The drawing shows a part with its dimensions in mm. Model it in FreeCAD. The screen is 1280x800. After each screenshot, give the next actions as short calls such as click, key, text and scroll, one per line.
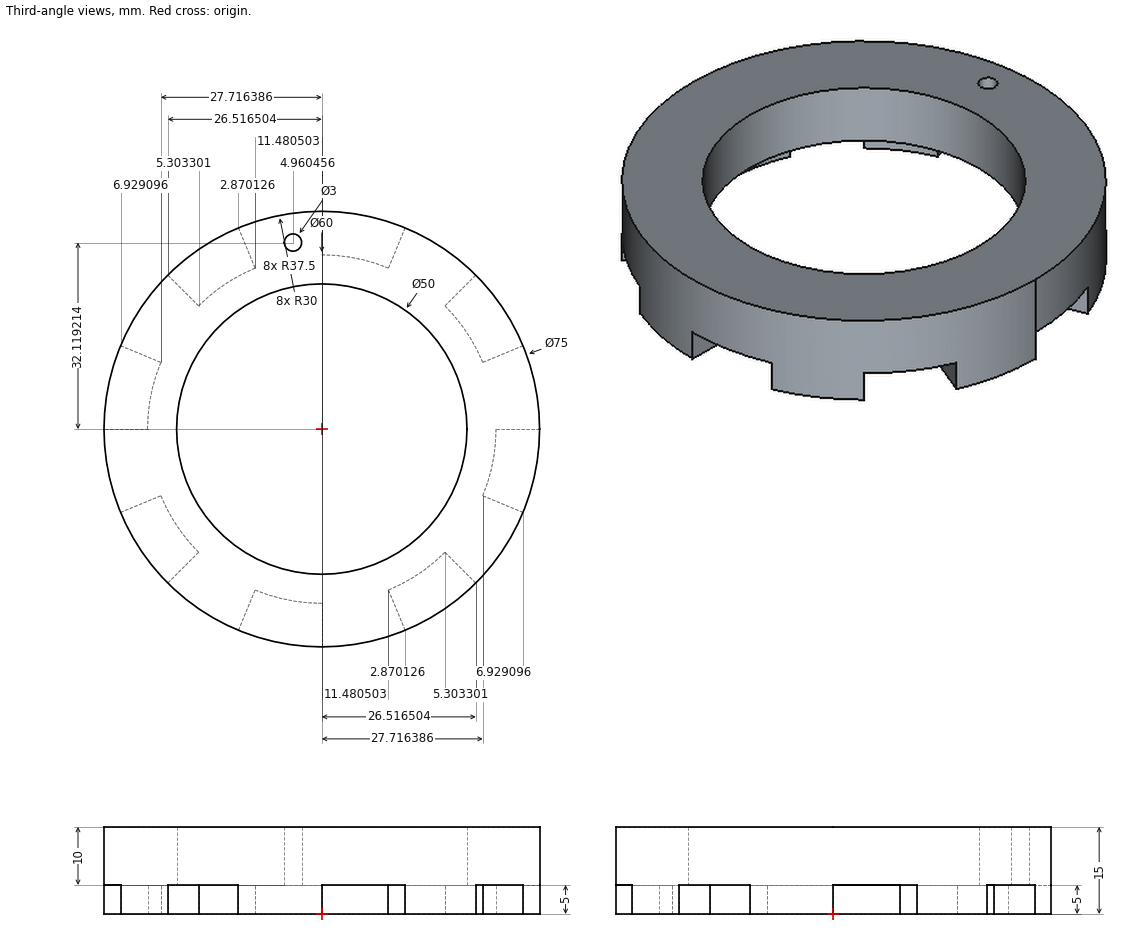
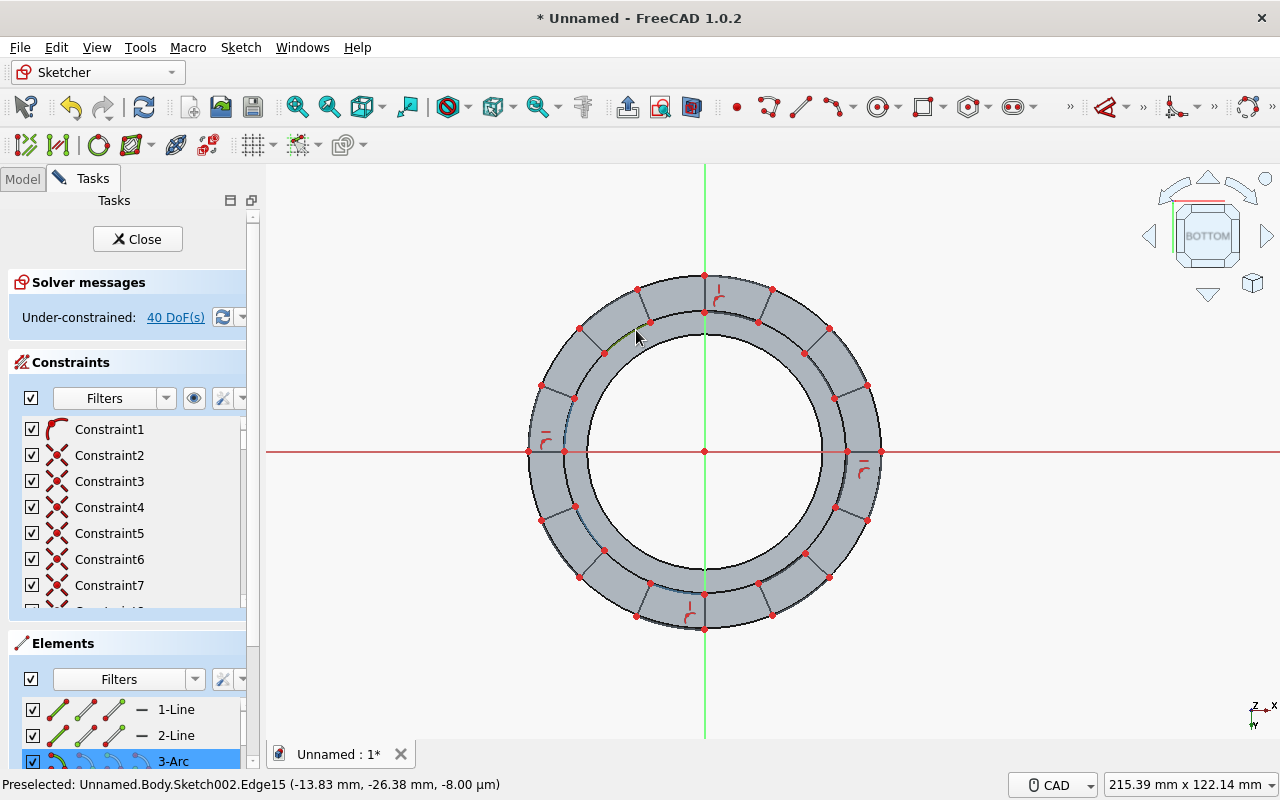
click(743, 318)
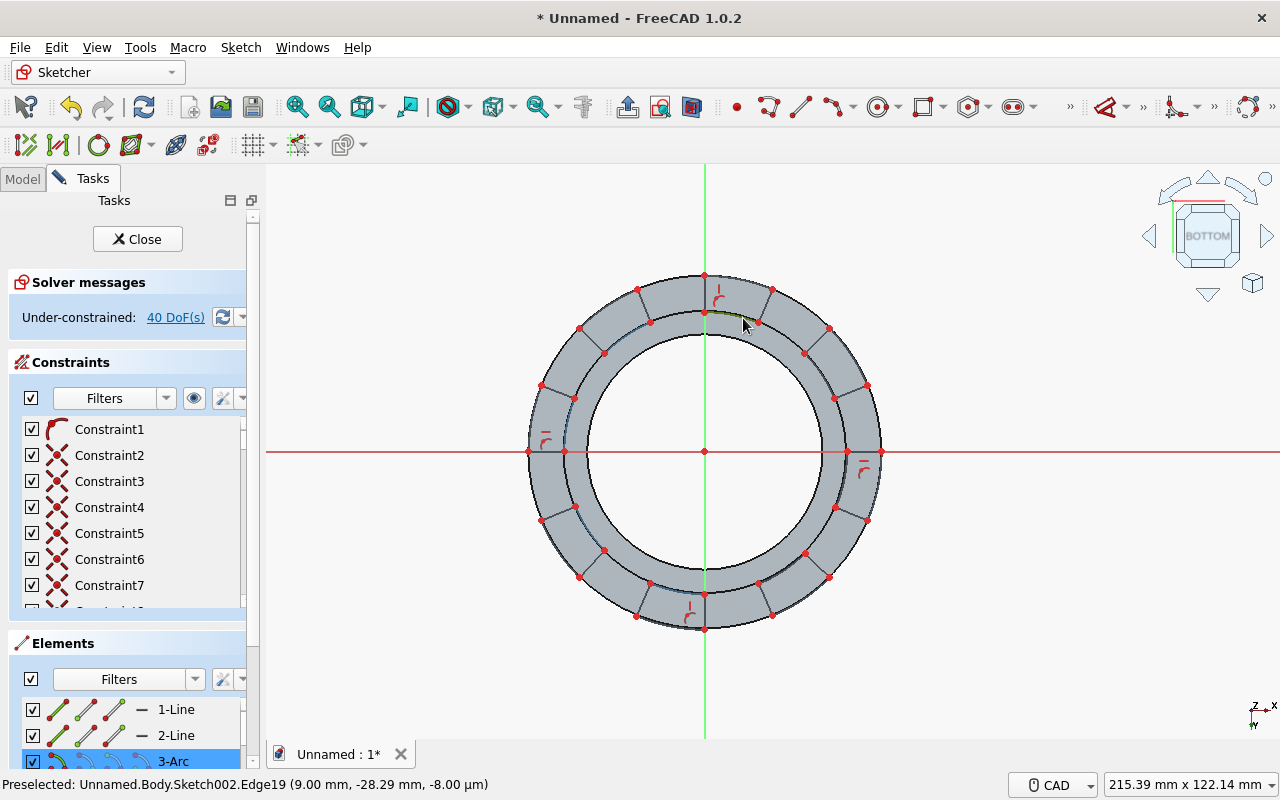
click(827, 384)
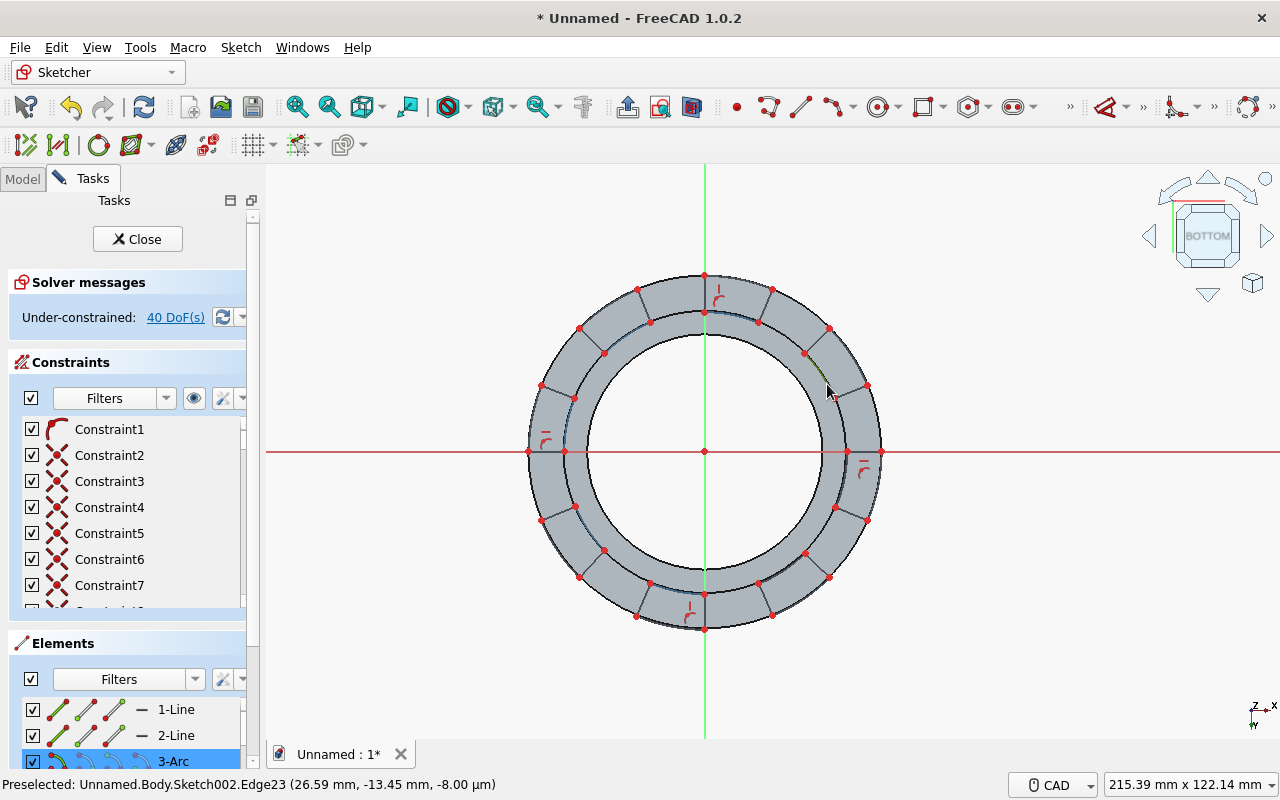
click(841, 491)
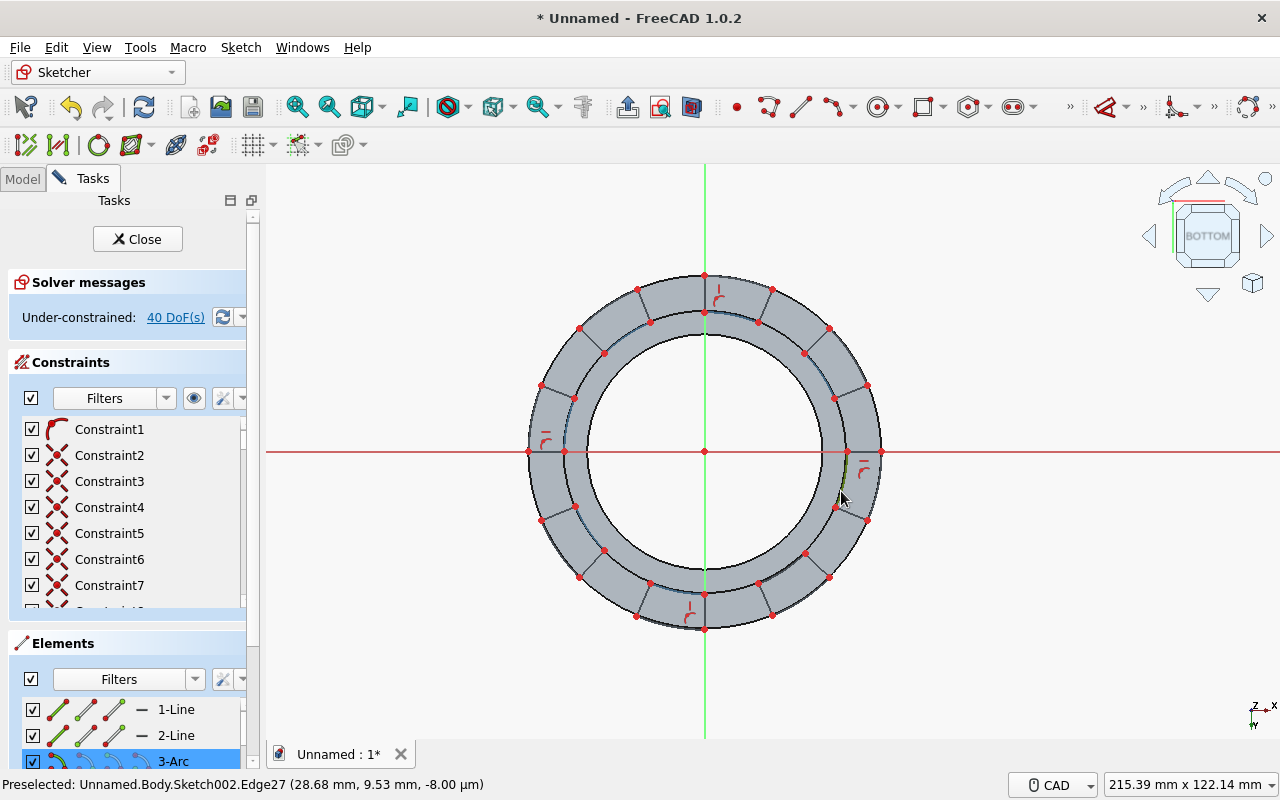
click(774, 577)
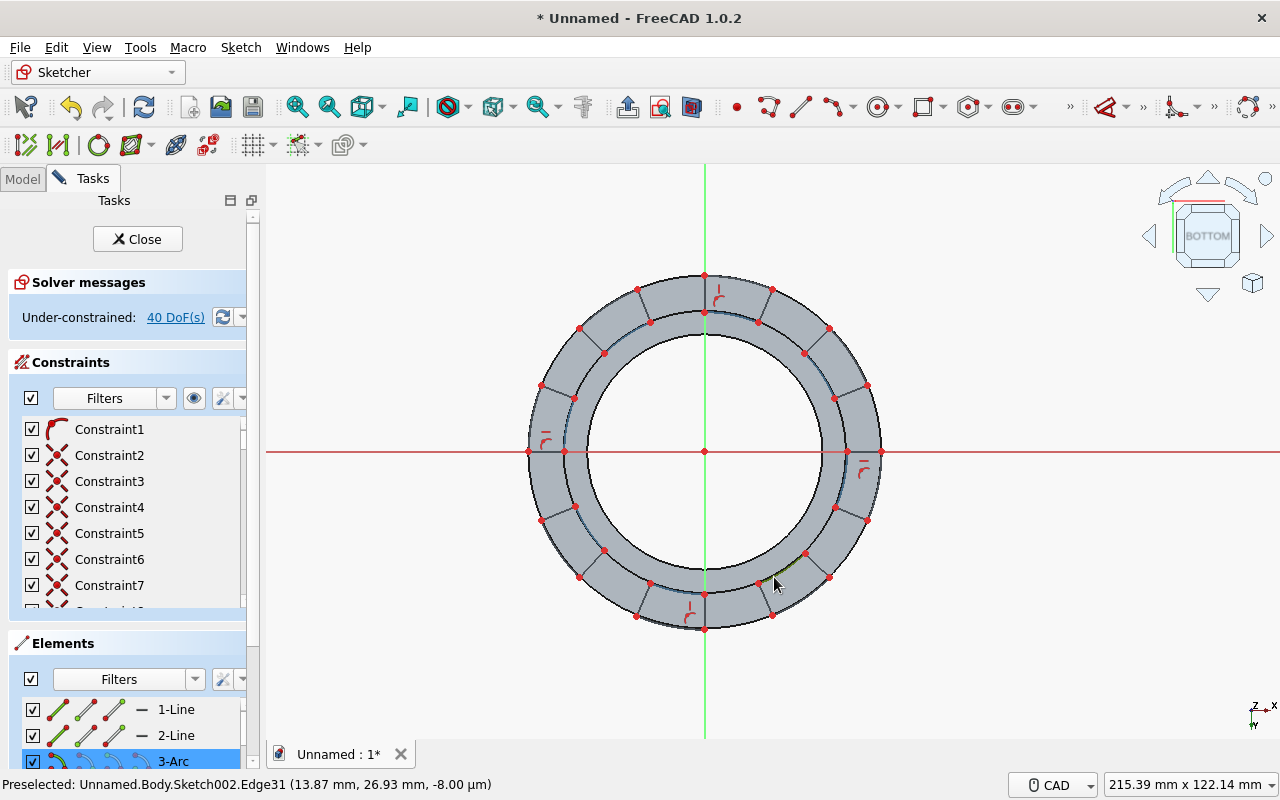
key(e)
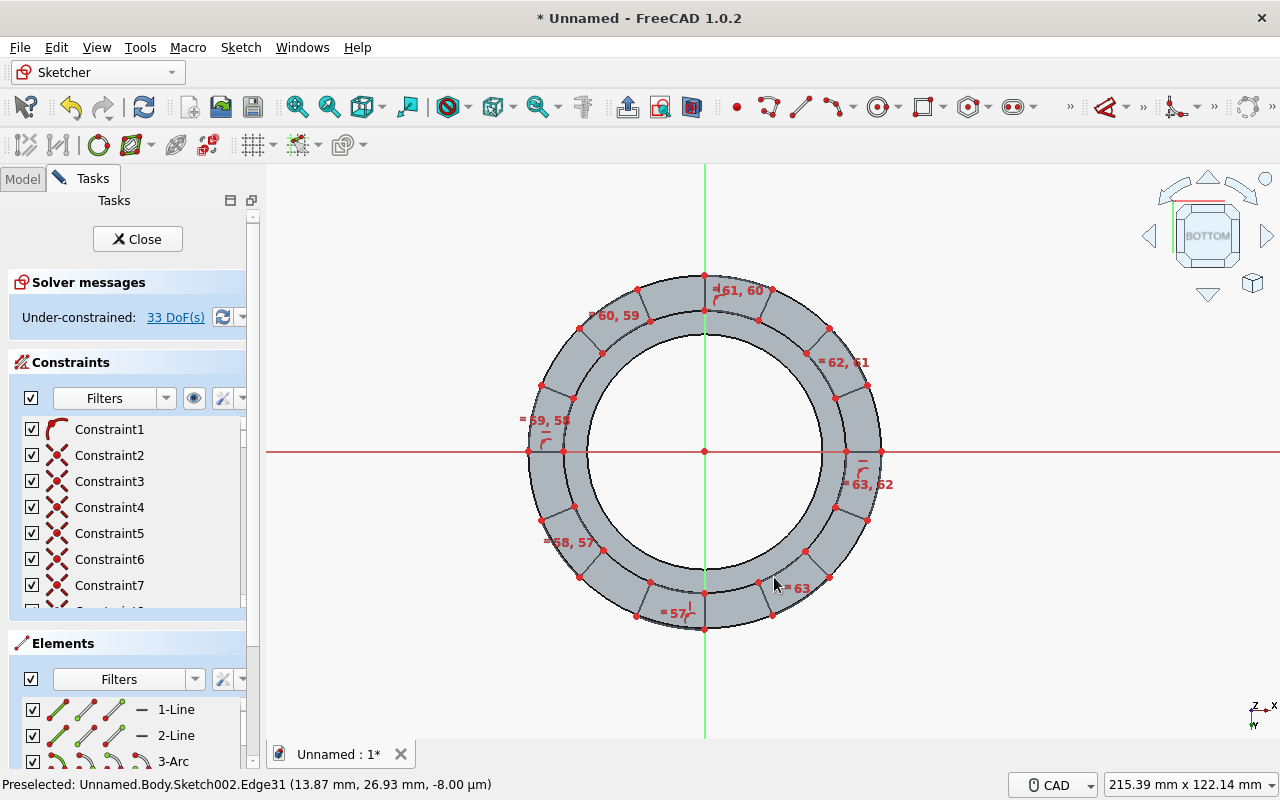
click(657, 623)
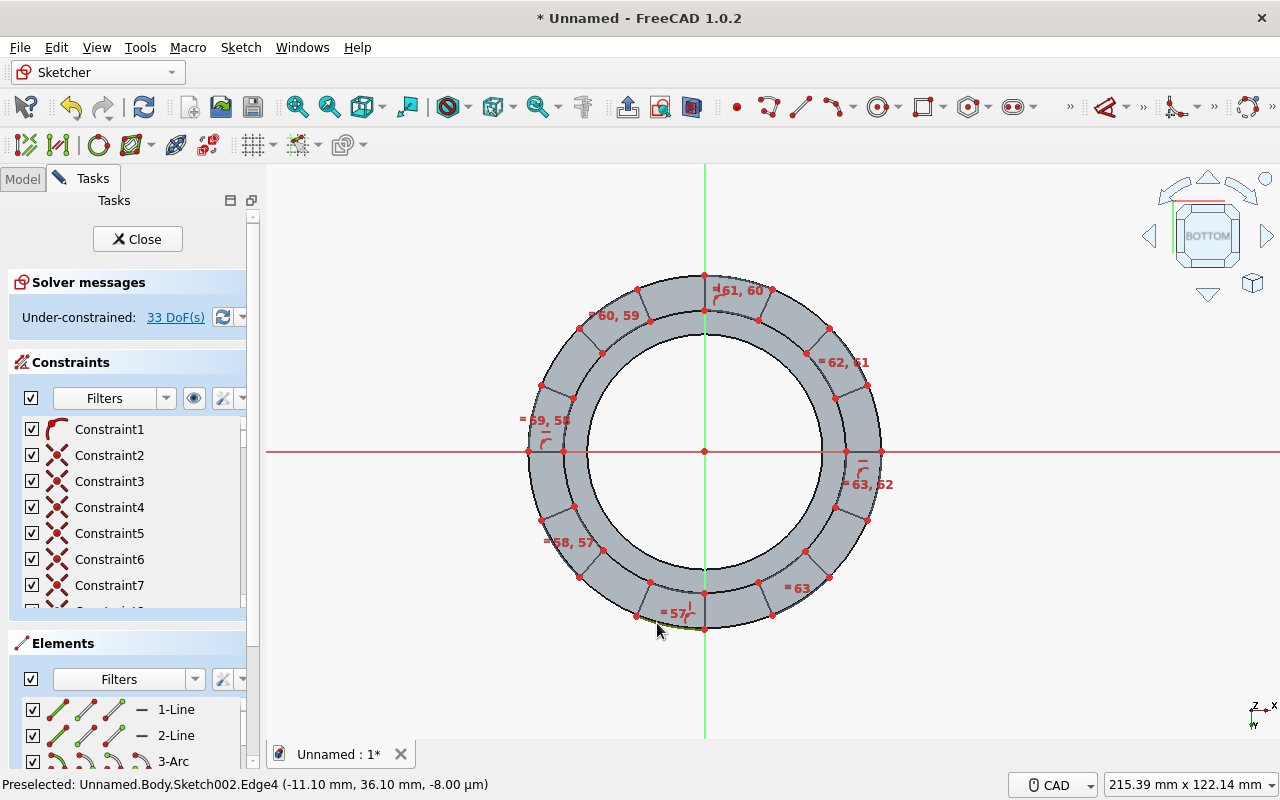
click(566, 562)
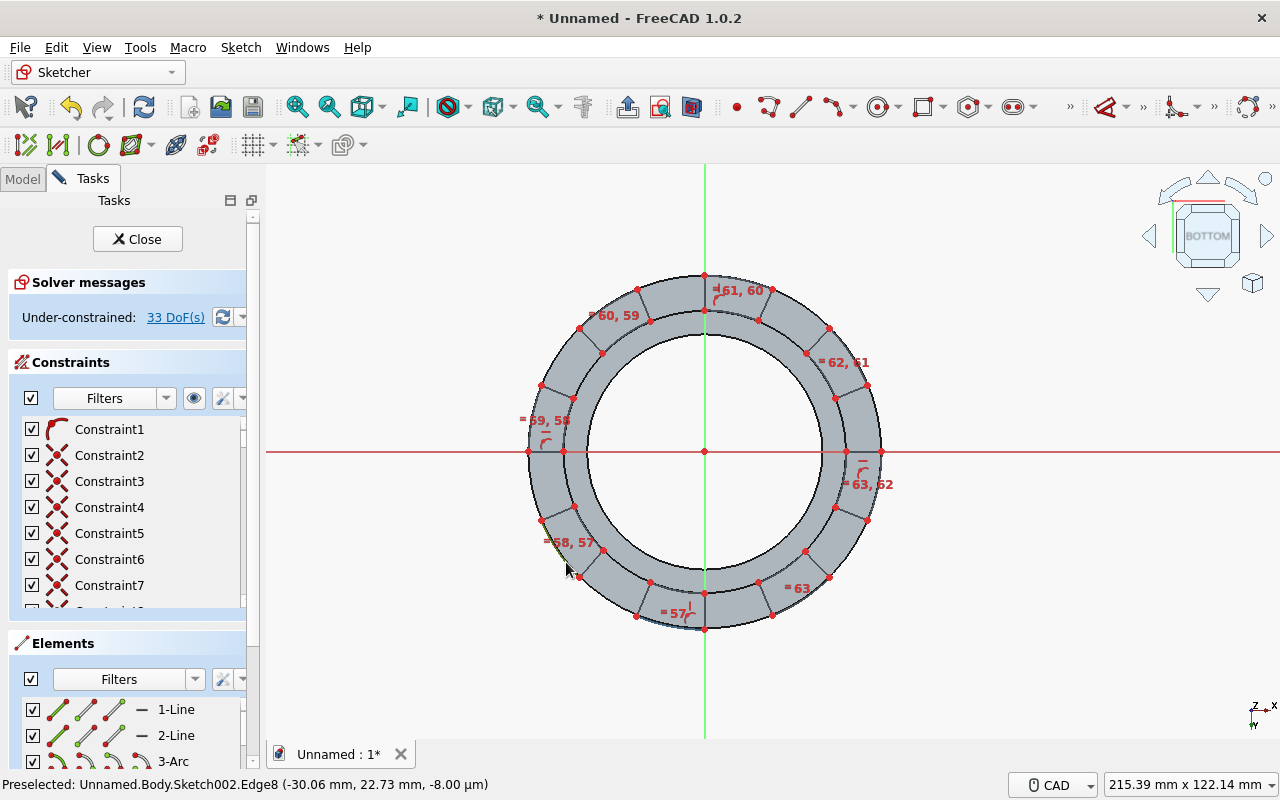
click(535, 405)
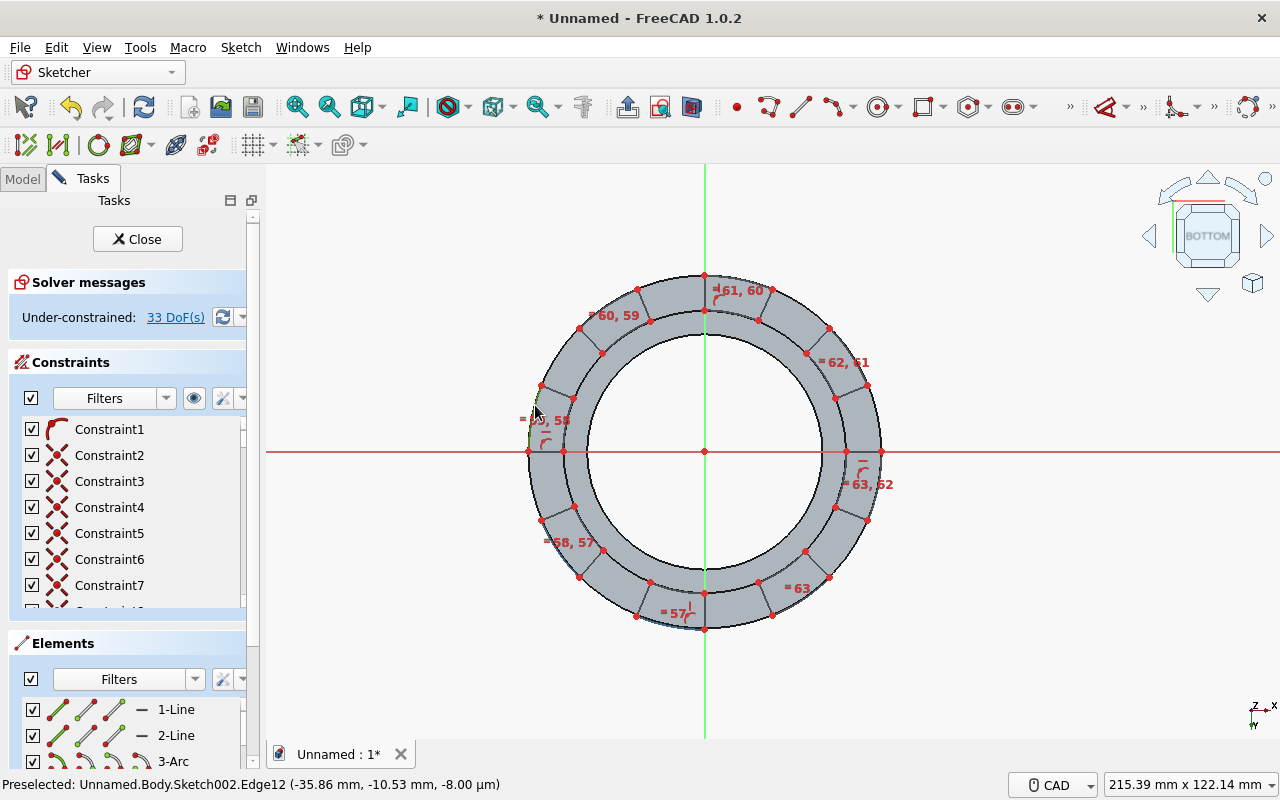
click(619, 299)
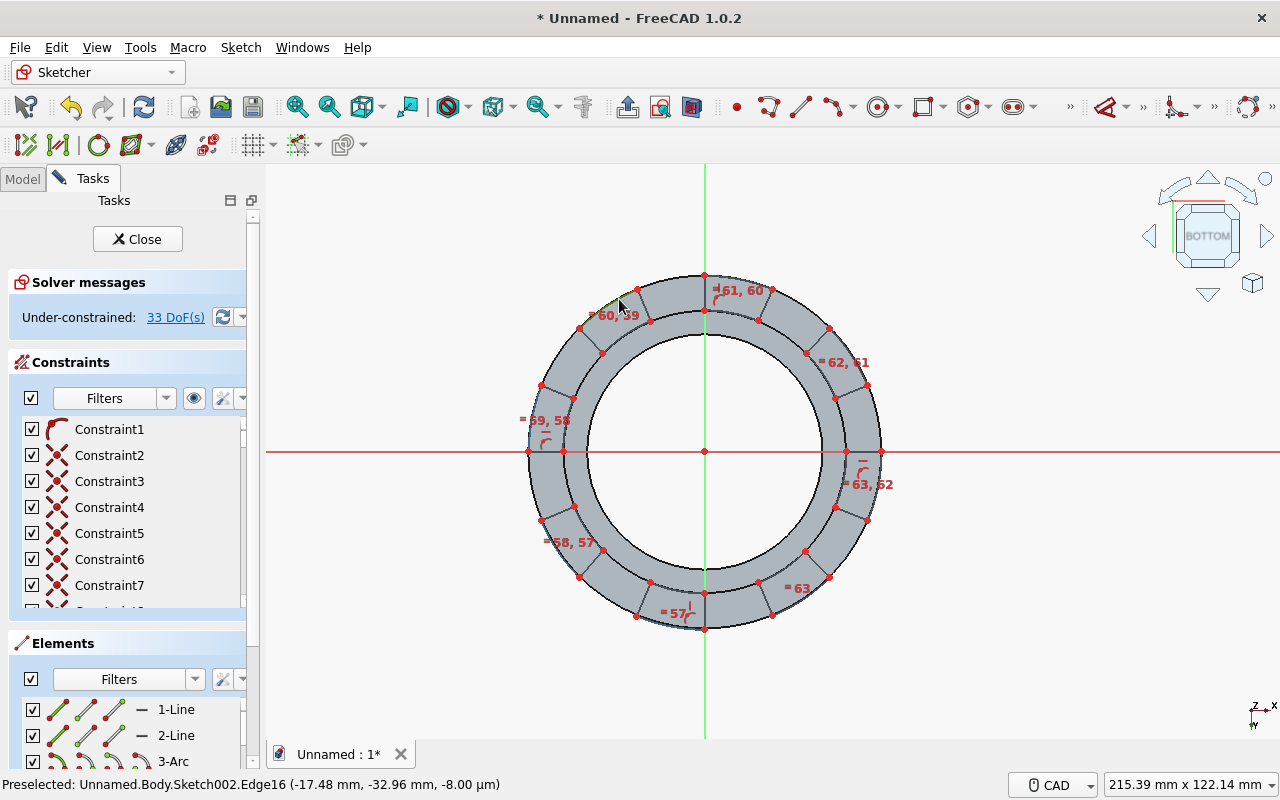
click(726, 277)